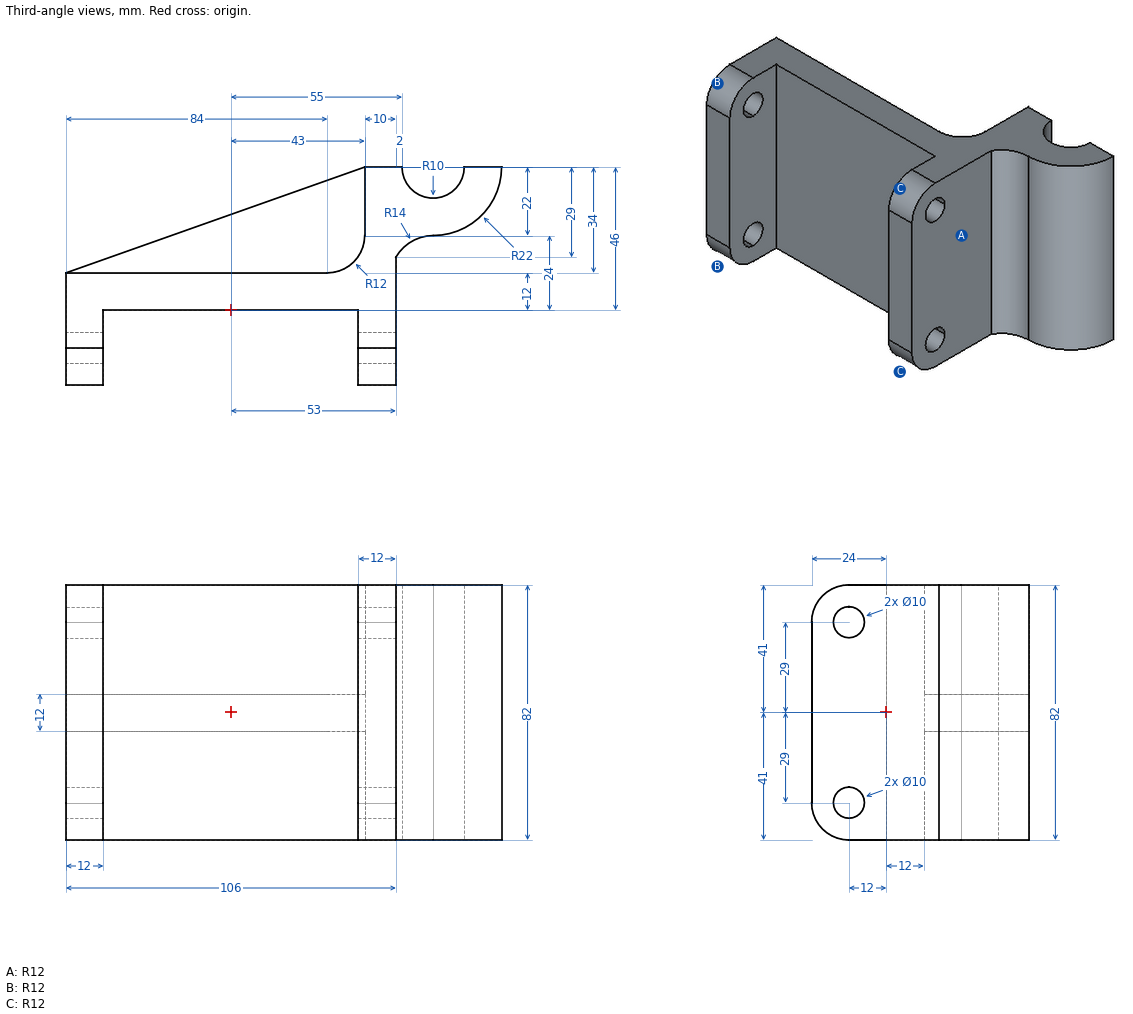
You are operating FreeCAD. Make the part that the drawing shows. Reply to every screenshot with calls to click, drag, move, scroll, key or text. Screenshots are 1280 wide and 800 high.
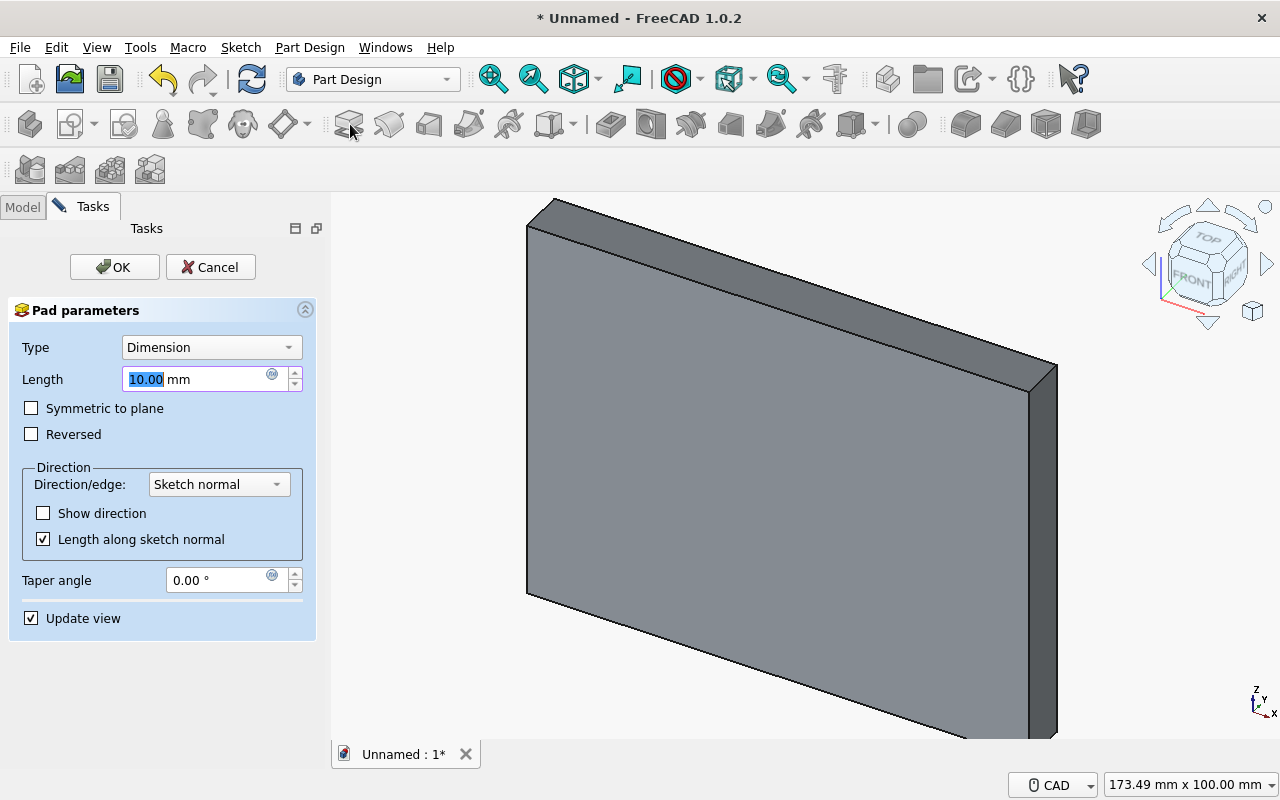
text(12)
key(Tab)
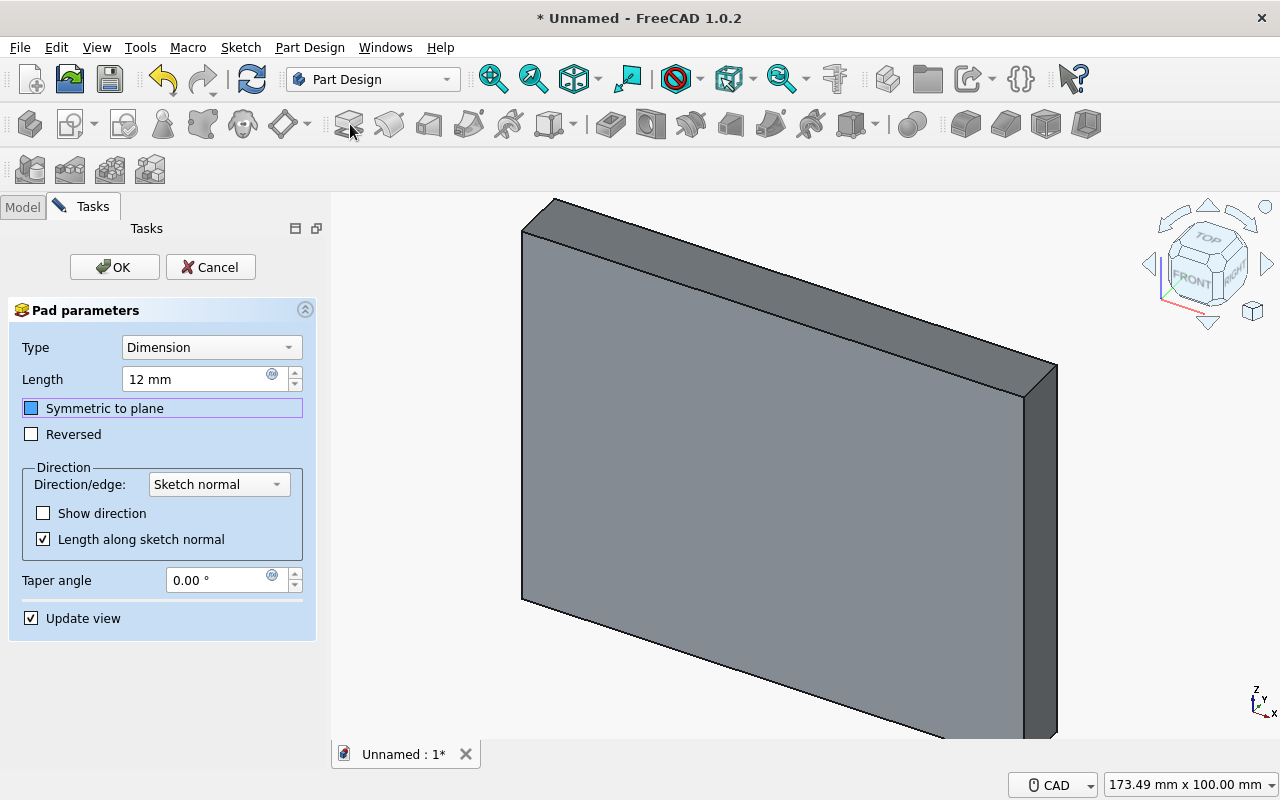
click(30, 434)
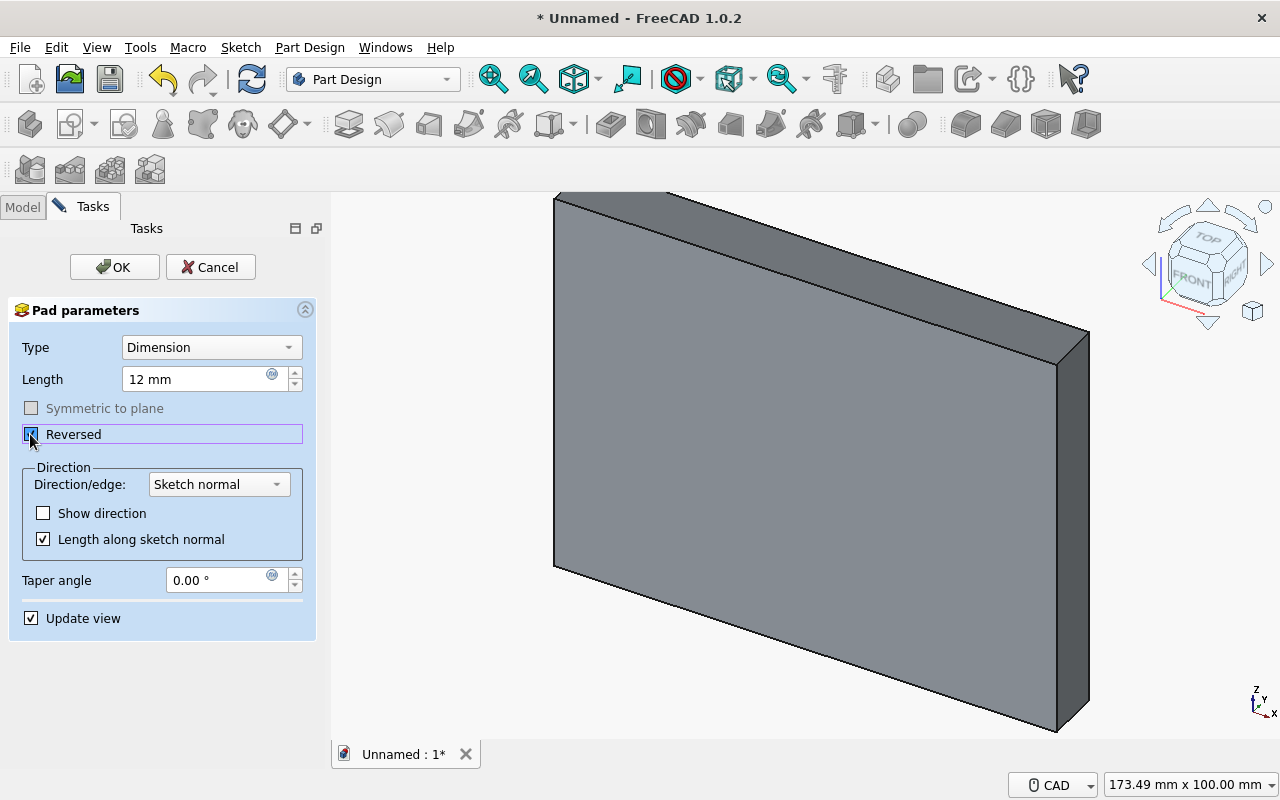
click(115, 267)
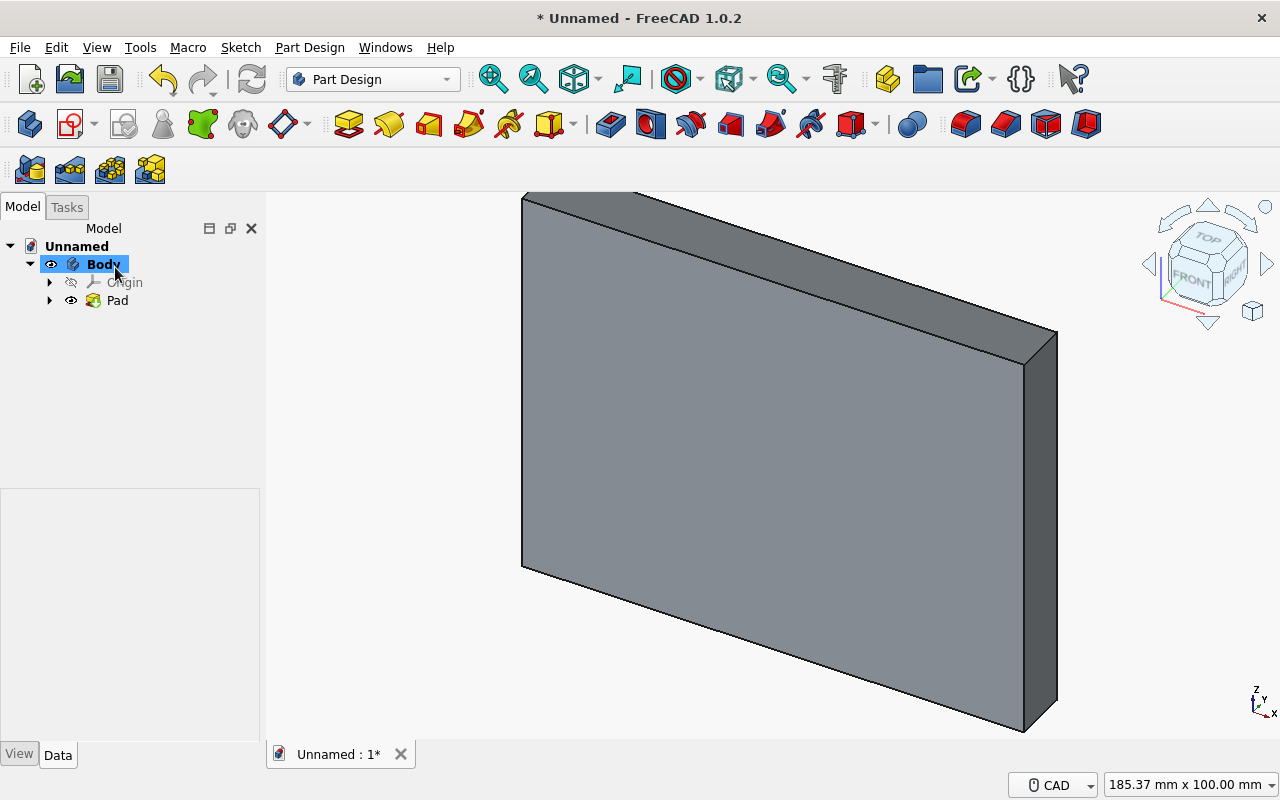
click(494, 80)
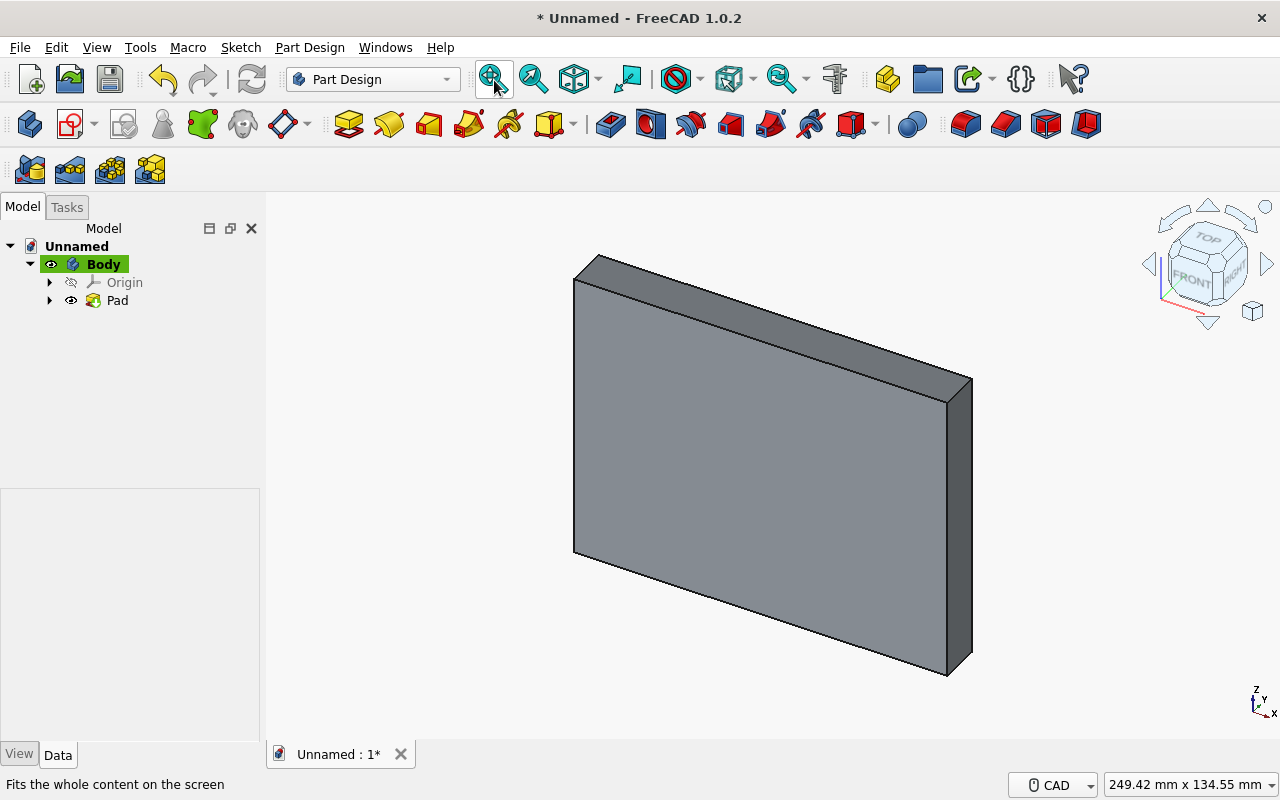
click(933, 381)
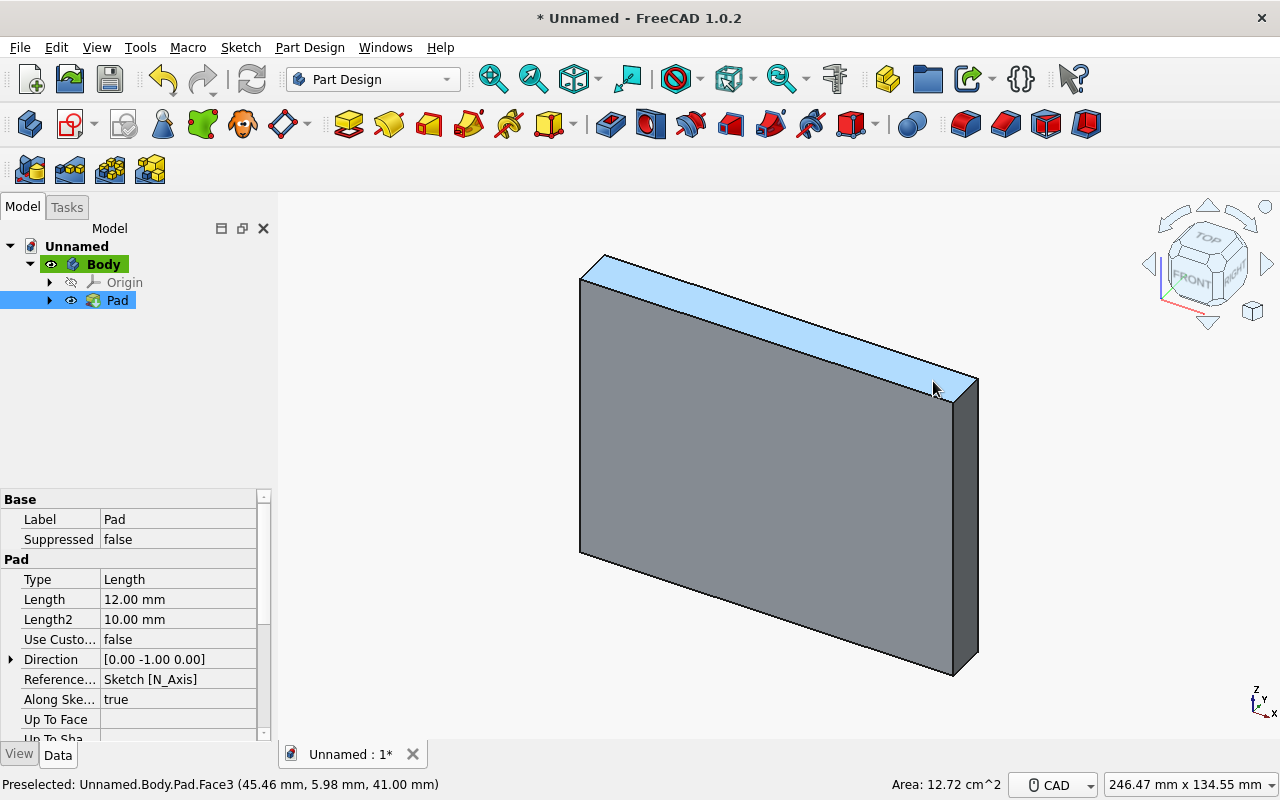
click(70, 124)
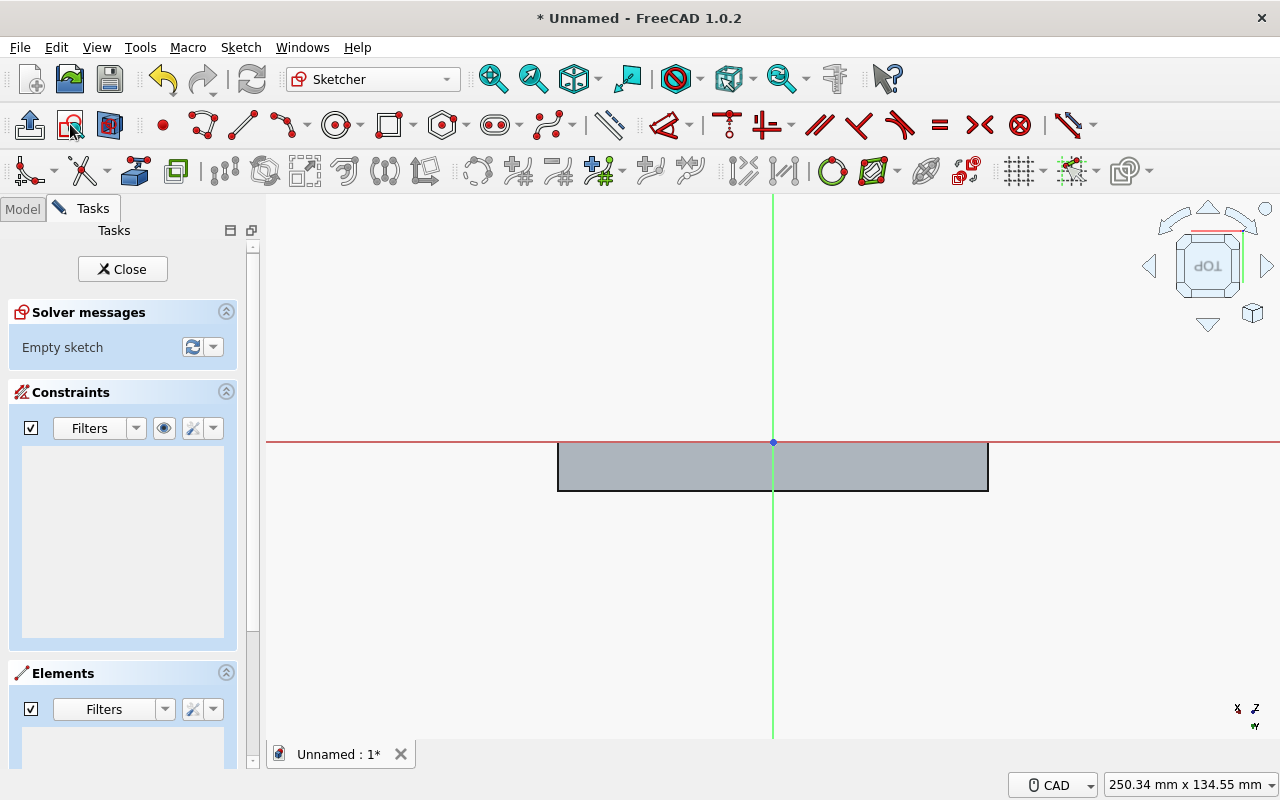
scroll(618, 619, up, 3)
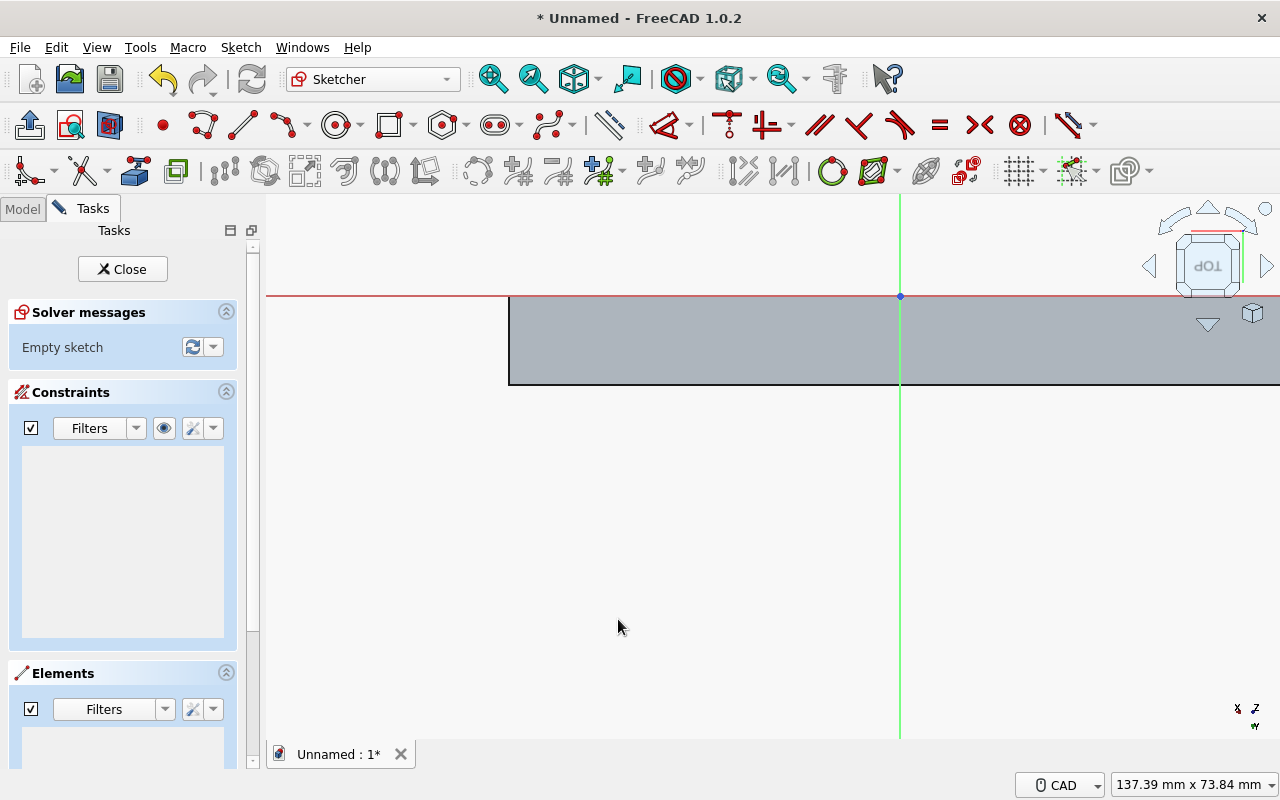
click(390, 126)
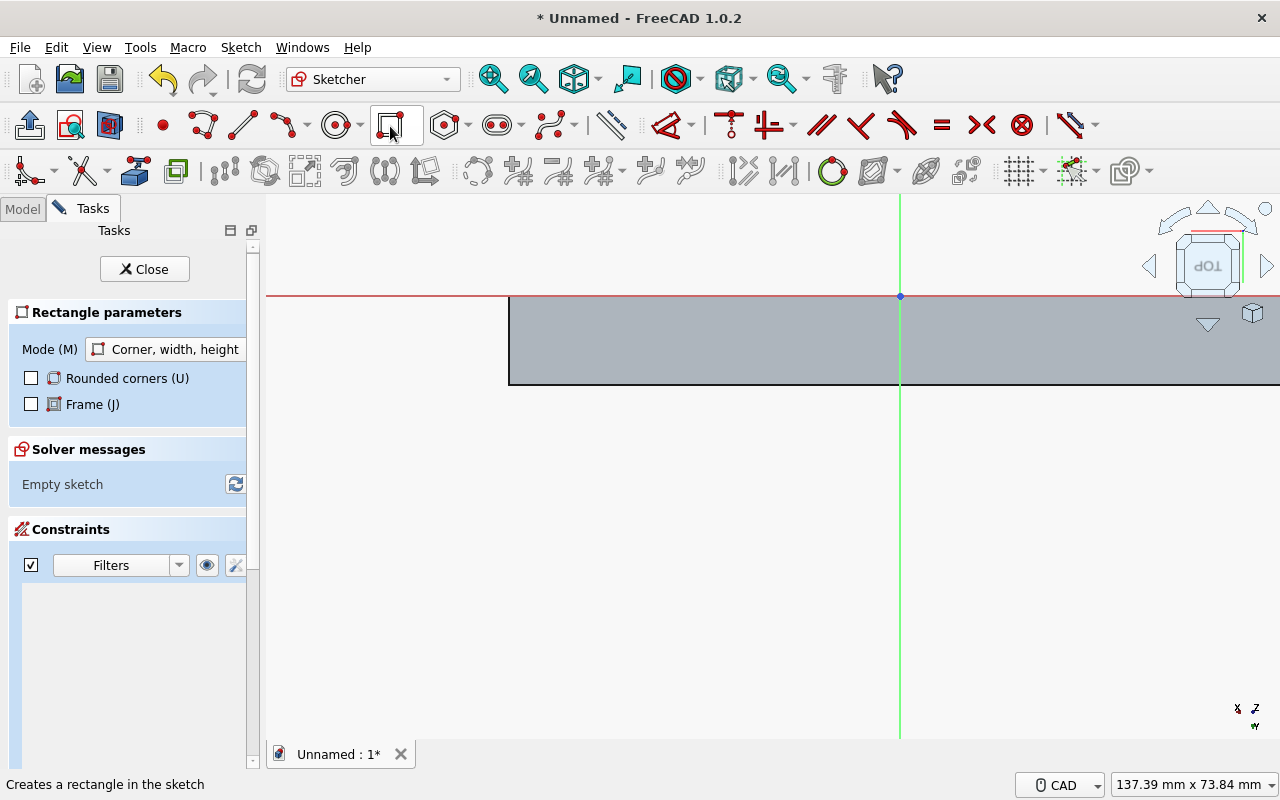
click(509, 385)
move(583, 636)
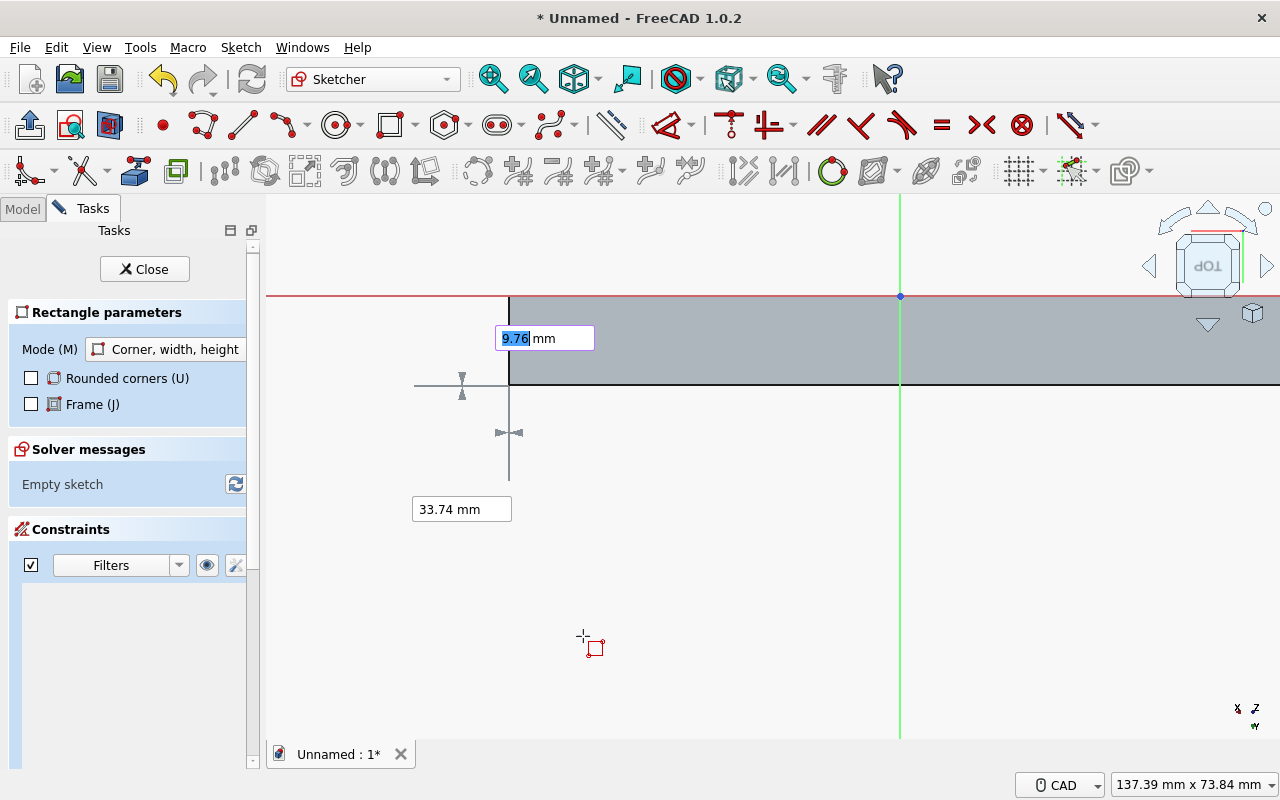
text(10)
key(Tab)
text(34)
key(Return)
key(Escape)